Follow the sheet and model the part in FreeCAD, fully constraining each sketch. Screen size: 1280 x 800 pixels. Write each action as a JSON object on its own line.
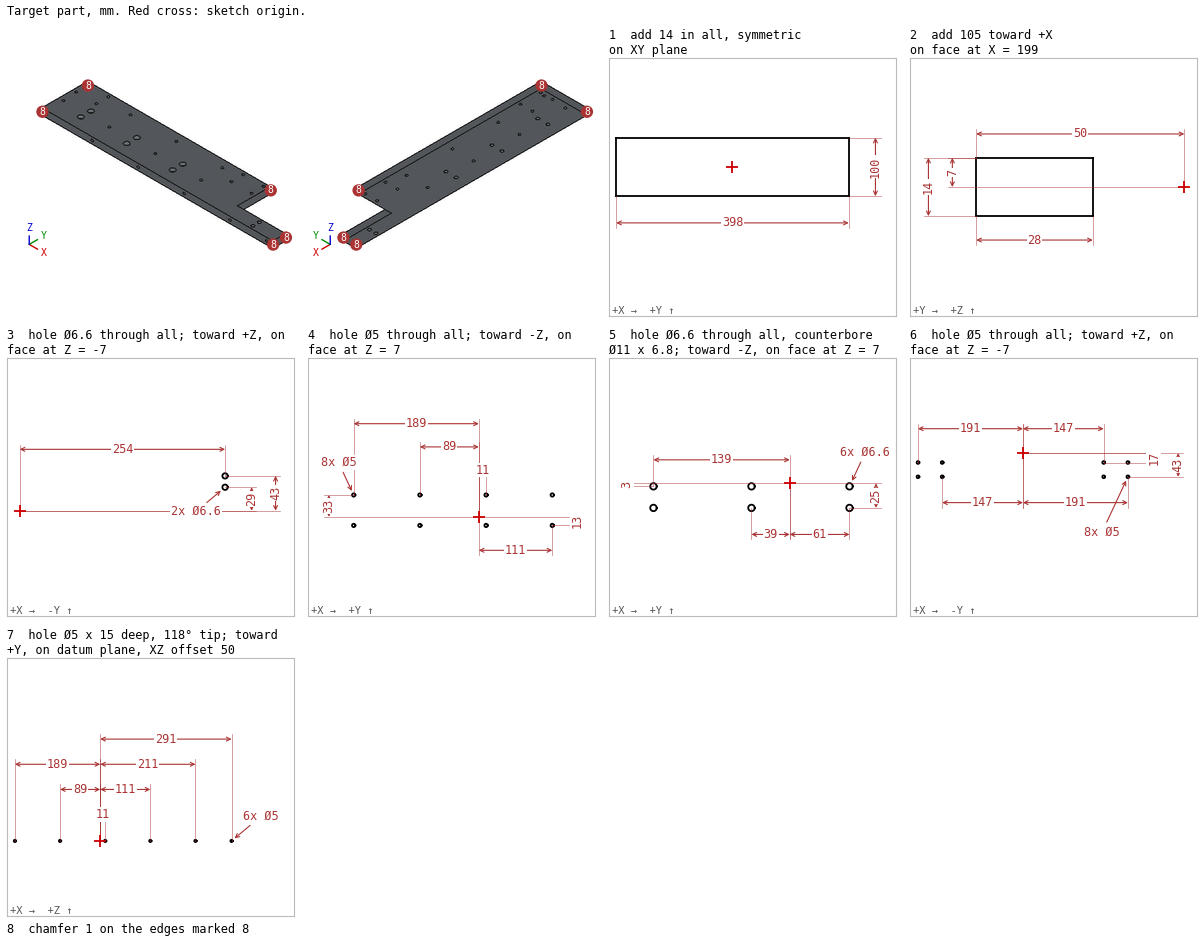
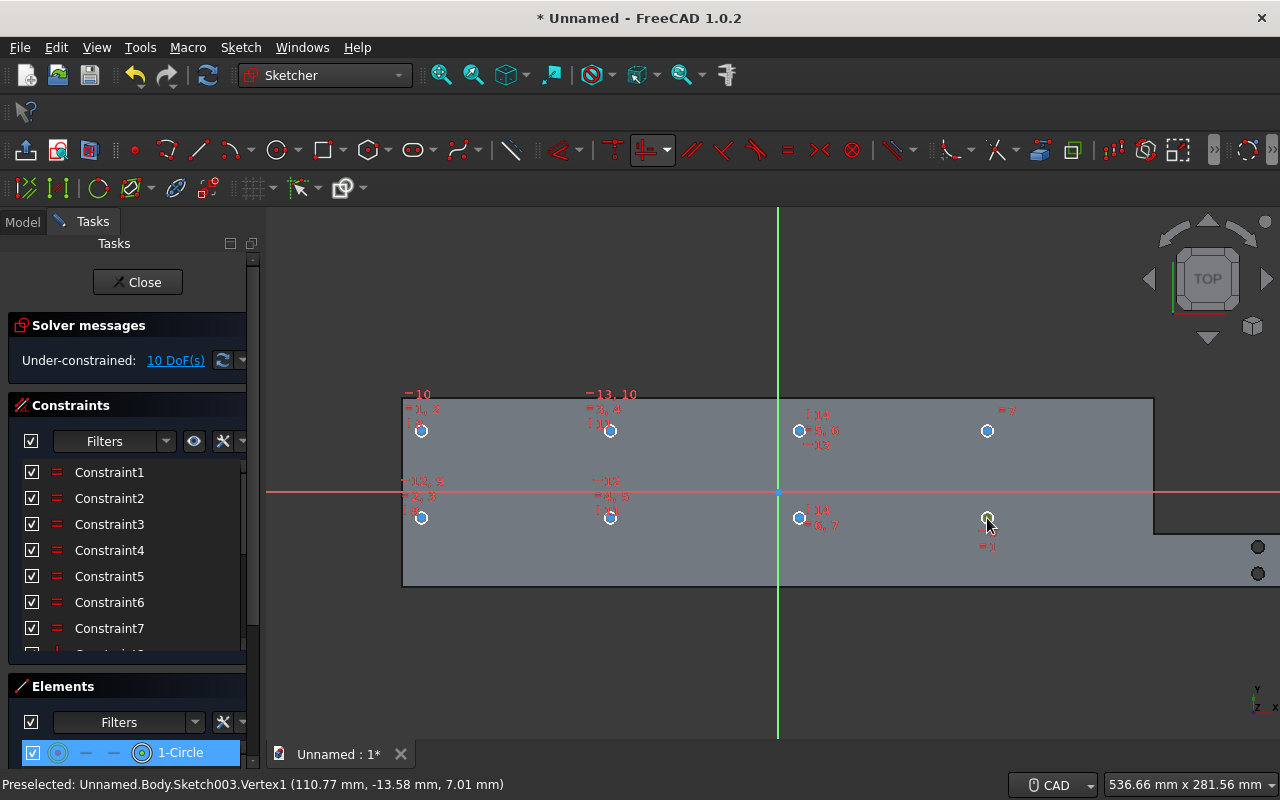
{"action": "left_click", "coordinate": [799, 518]}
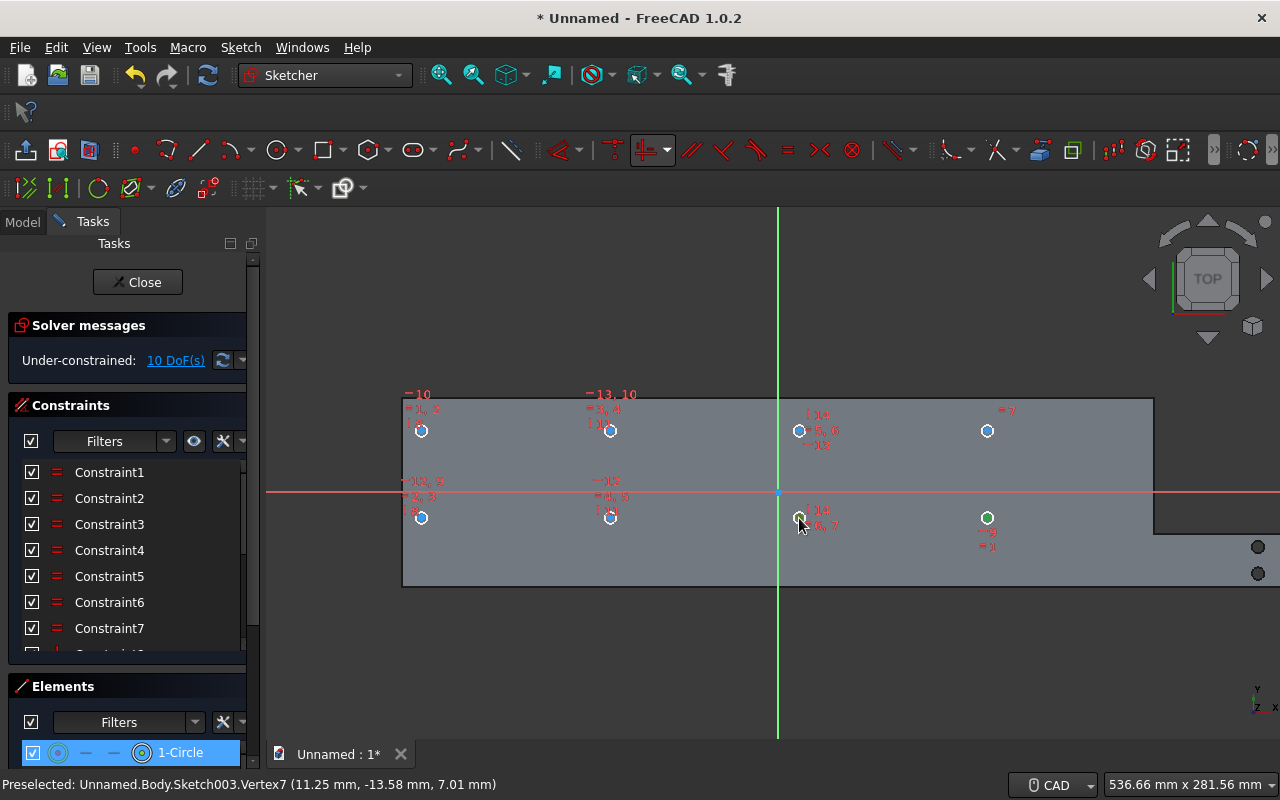
{"action": "key", "text": "h"}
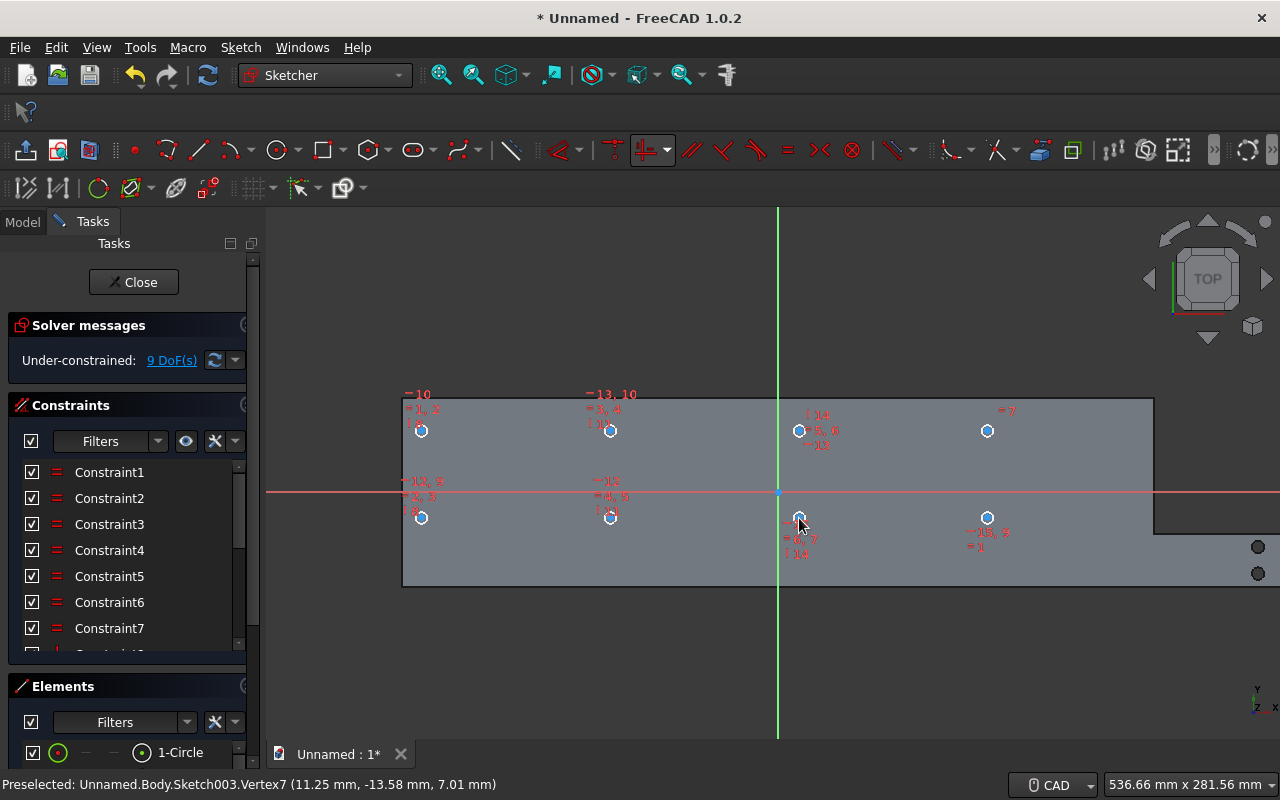
{"action": "left_click", "coordinate": [987, 518]}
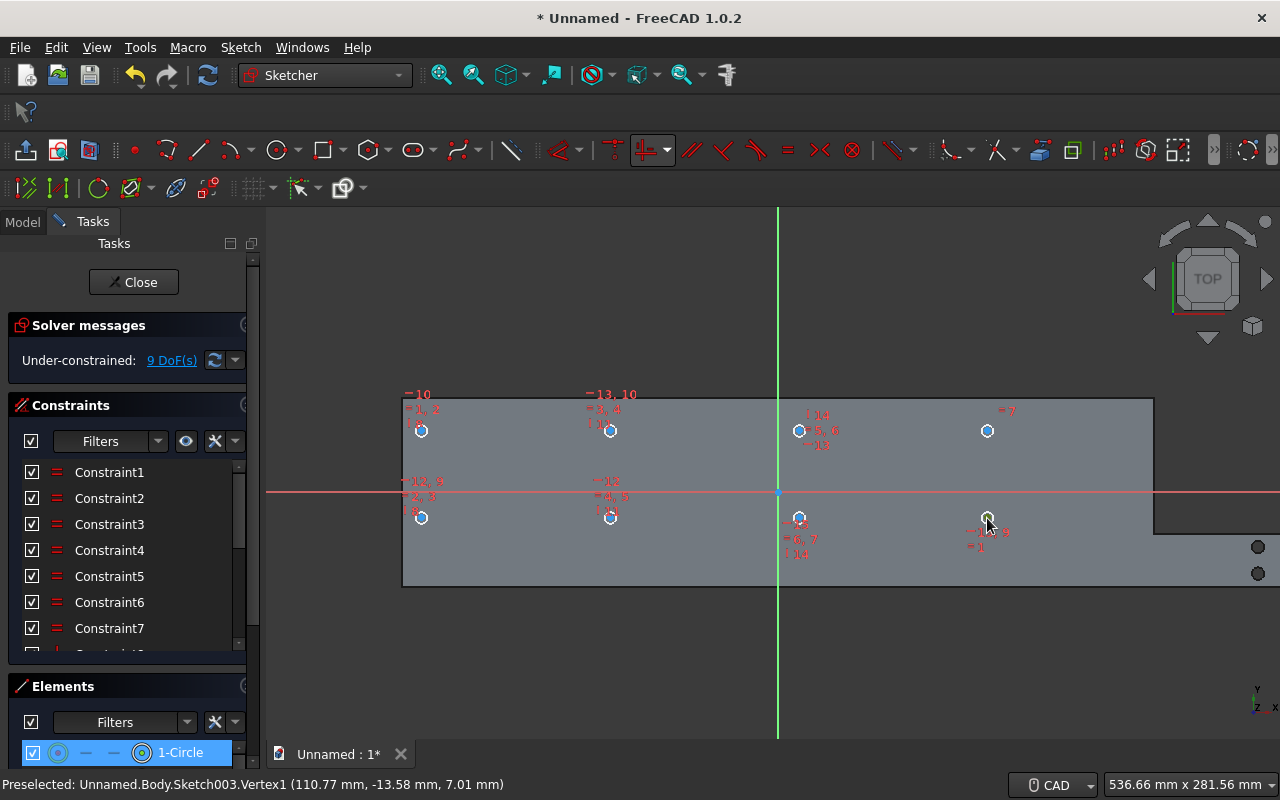
{"action": "left_click", "coordinate": [987, 431]}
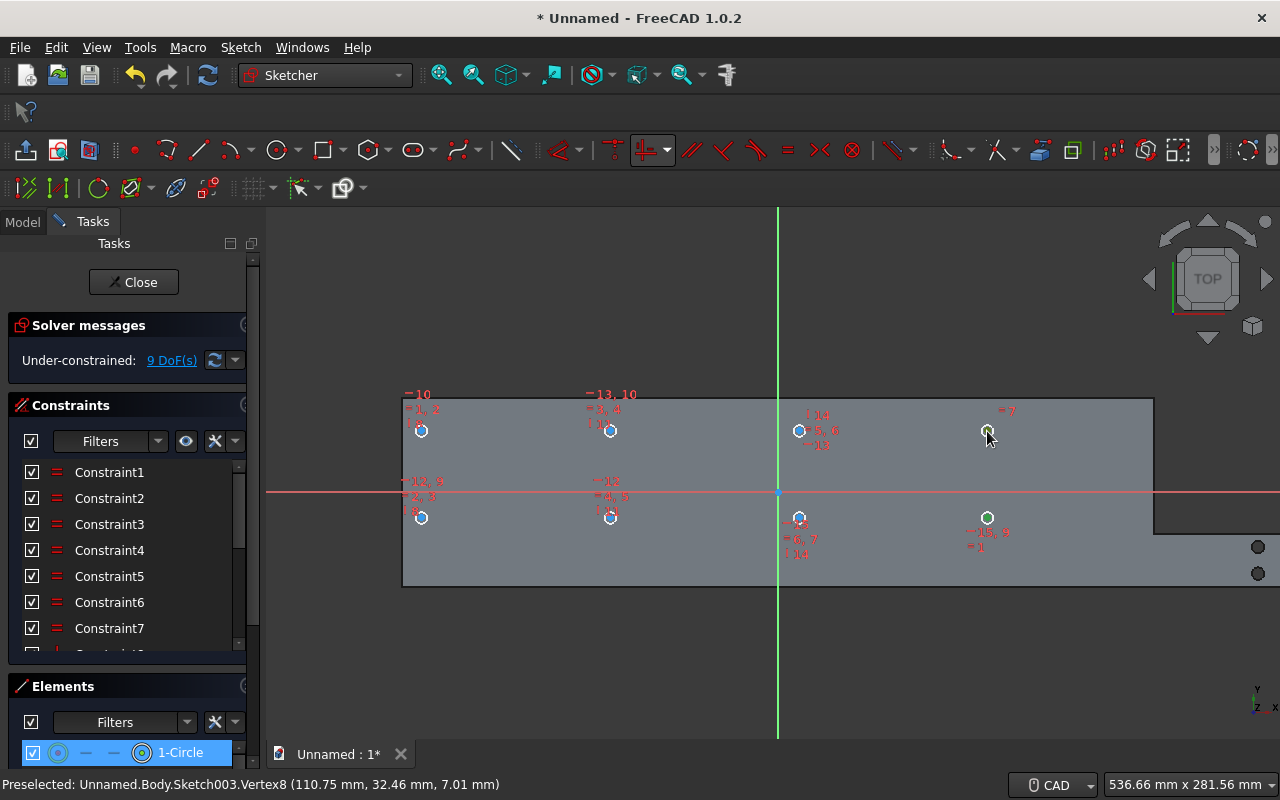
{"action": "key", "text": "v"}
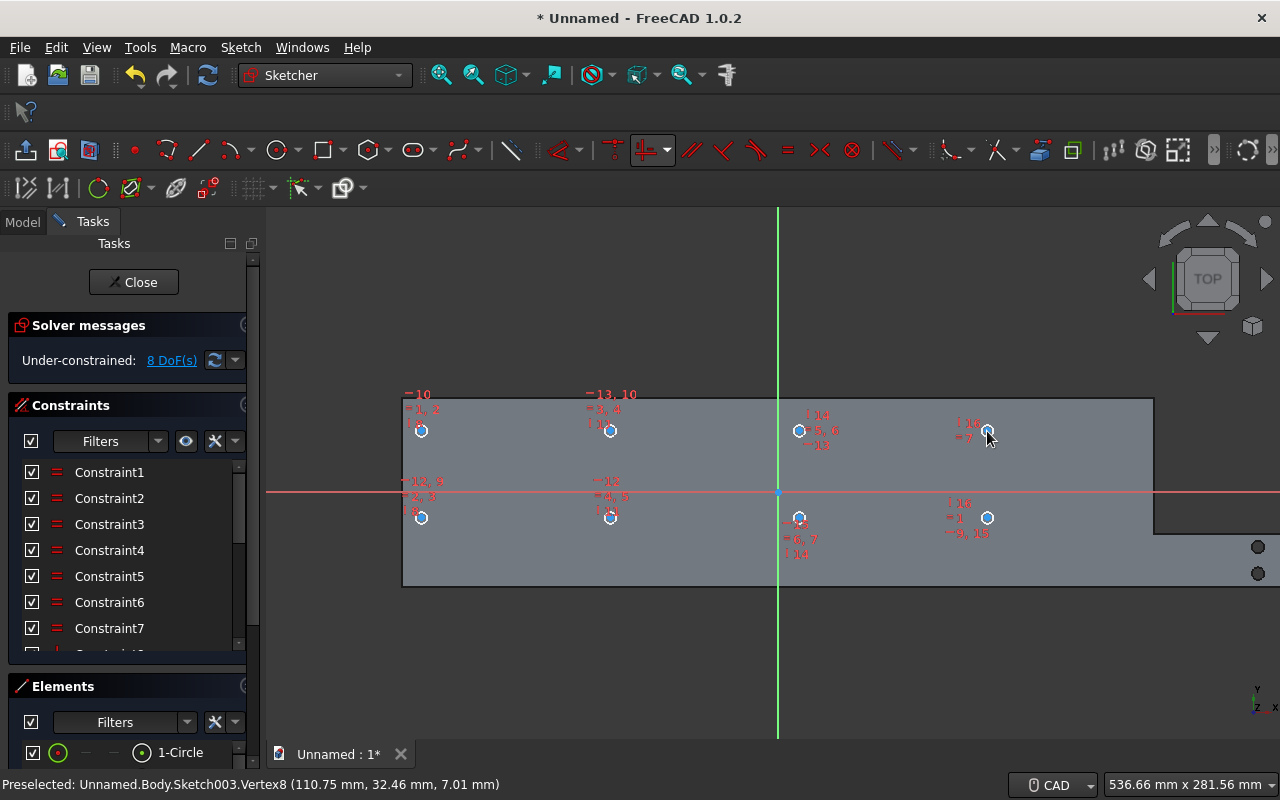
{"action": "left_click", "coordinate": [799, 431]}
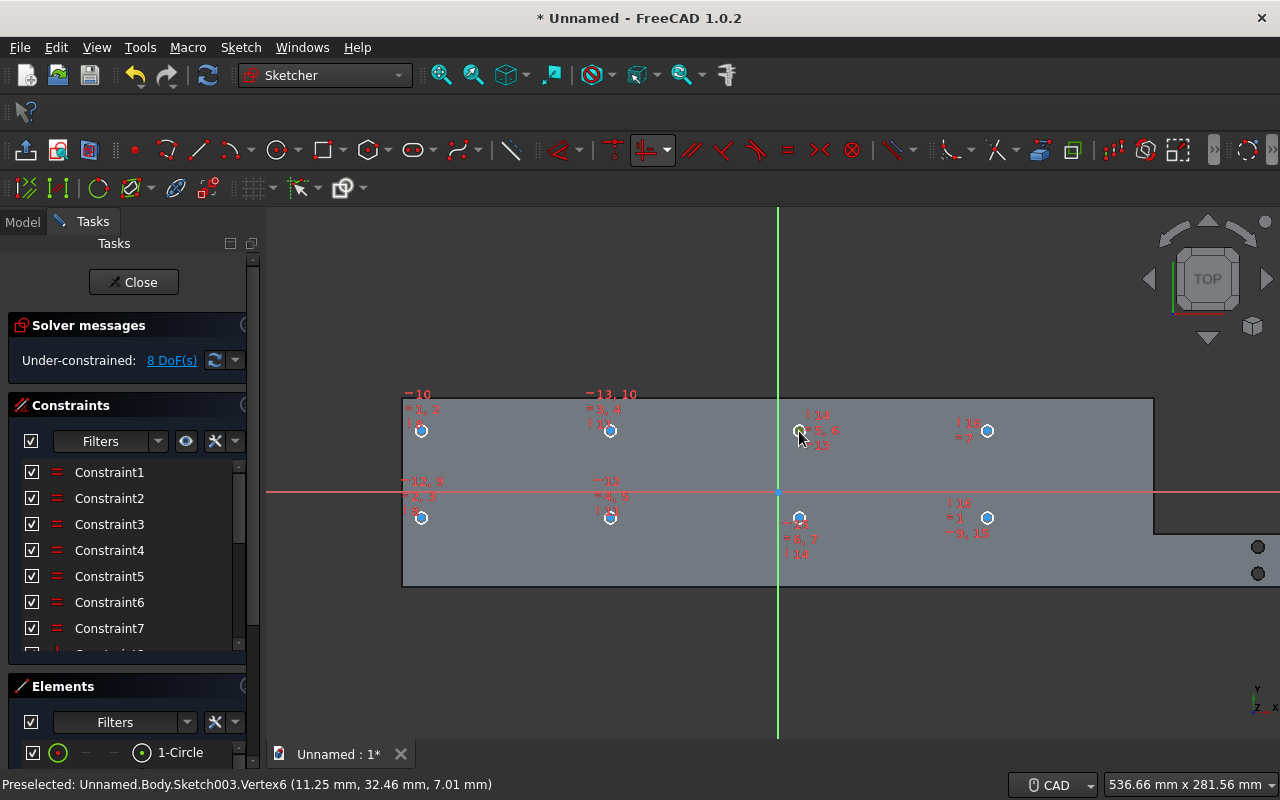
{"action": "left_click", "coordinate": [987, 431]}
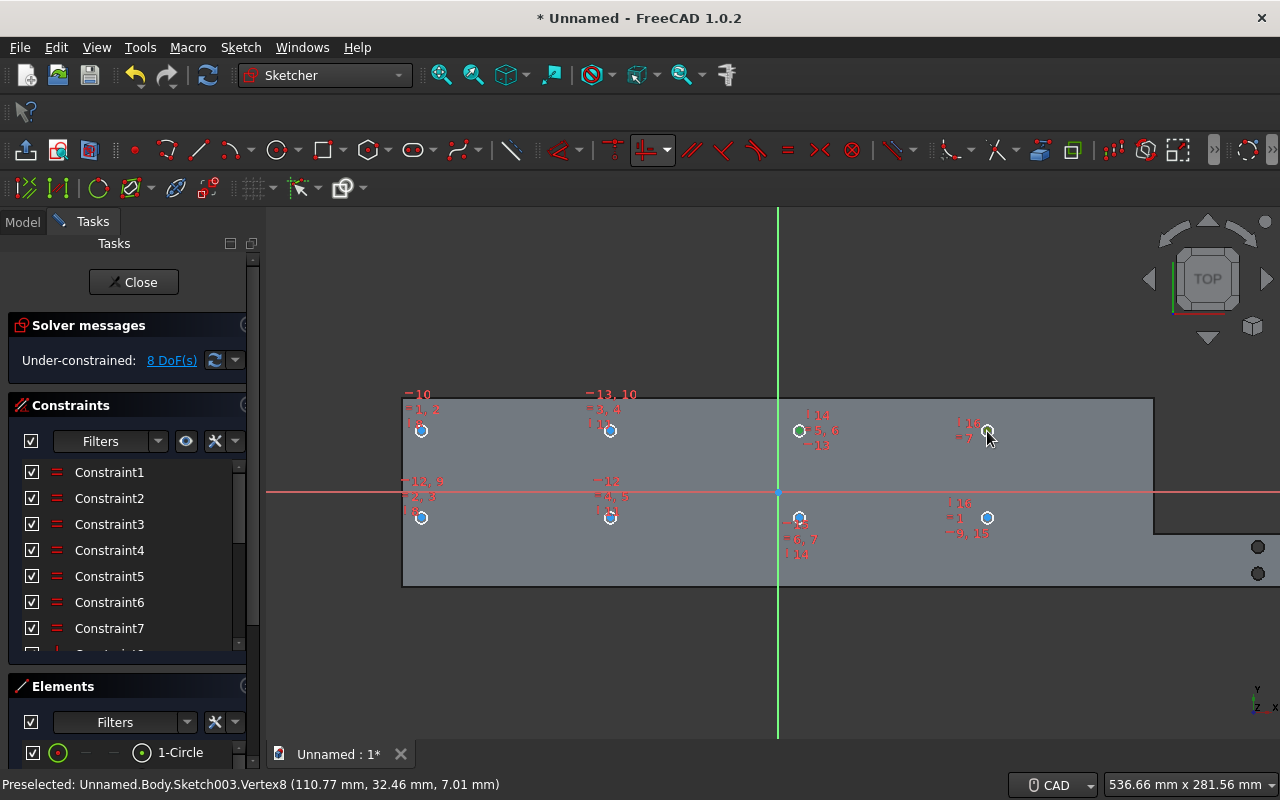
{"action": "key", "text": "h"}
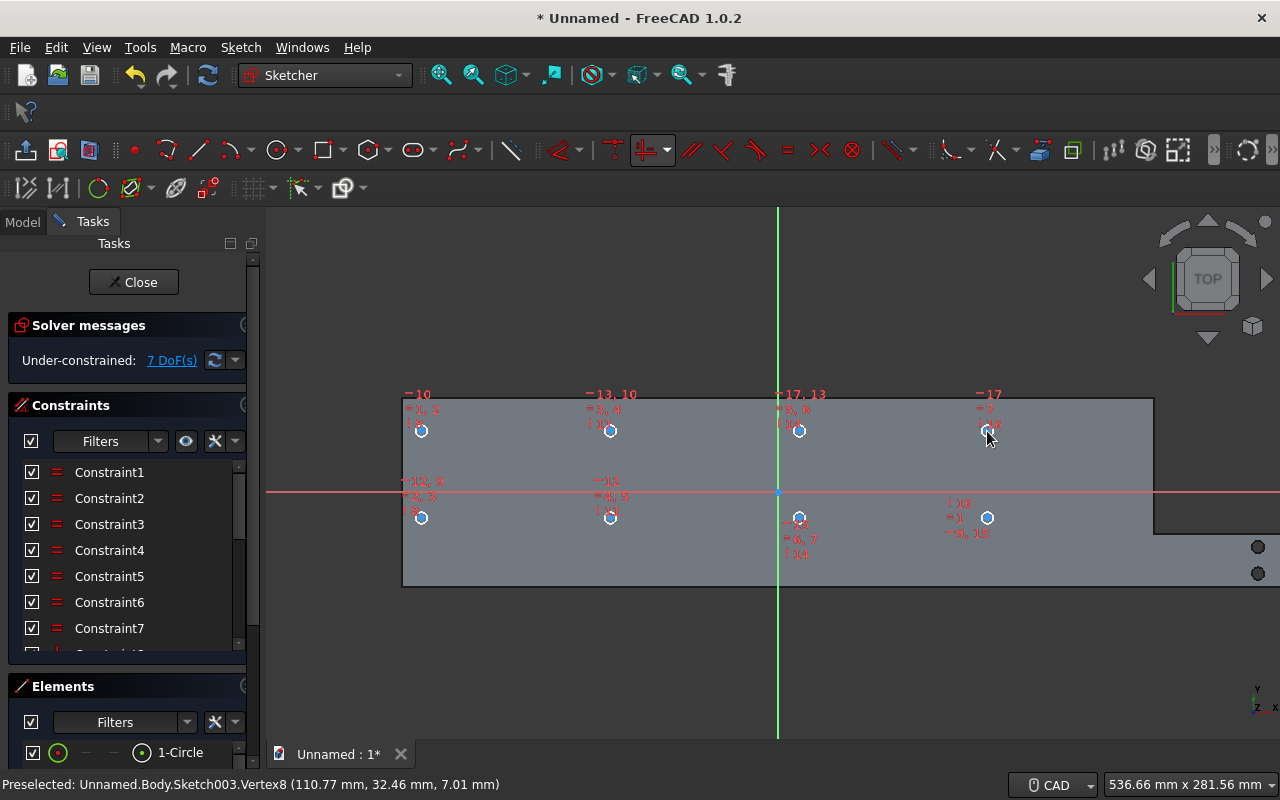
{"action": "left_click", "coordinate": [558, 150]}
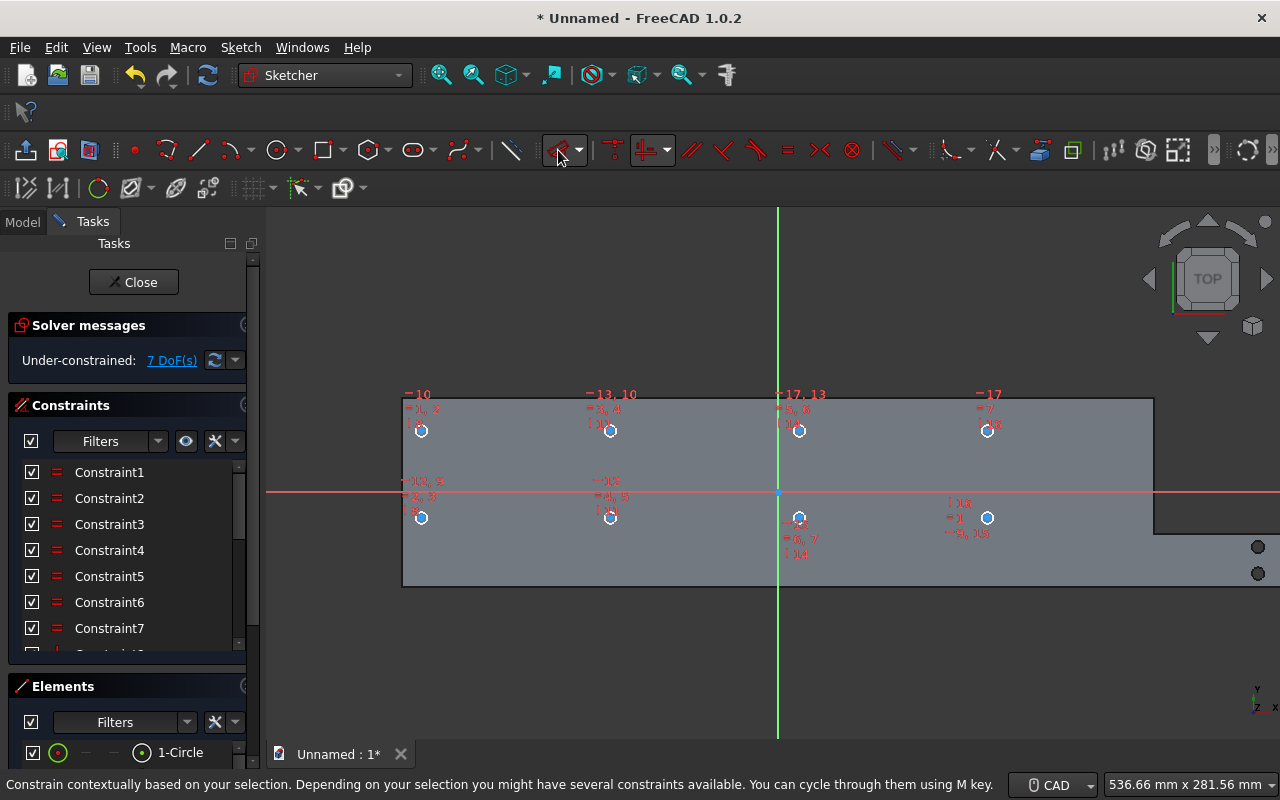
{"action": "scroll", "coordinate": [988, 512], "scroll_direction": "up", "scroll_amount": 8}